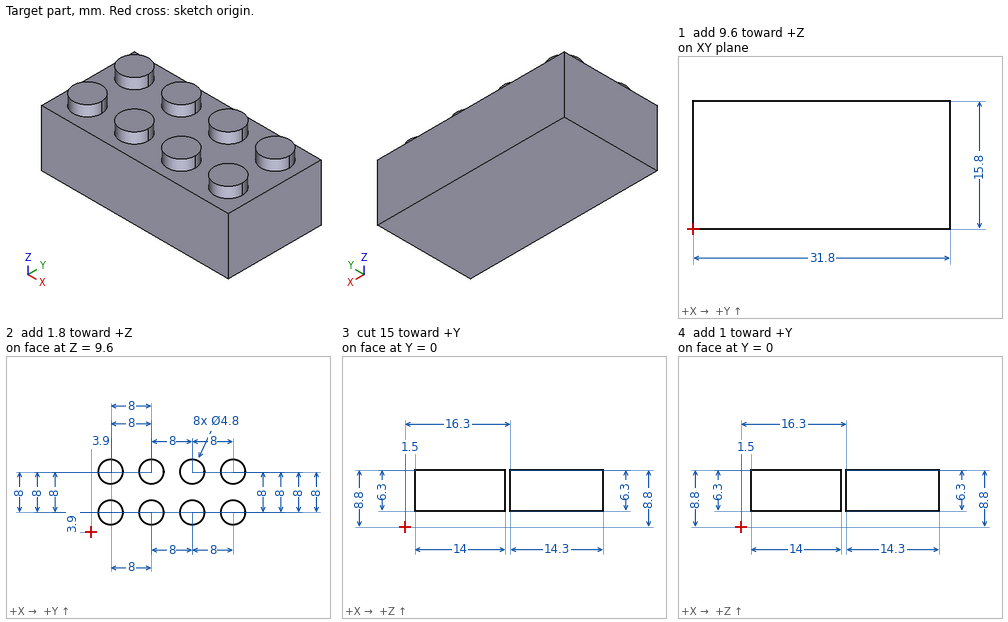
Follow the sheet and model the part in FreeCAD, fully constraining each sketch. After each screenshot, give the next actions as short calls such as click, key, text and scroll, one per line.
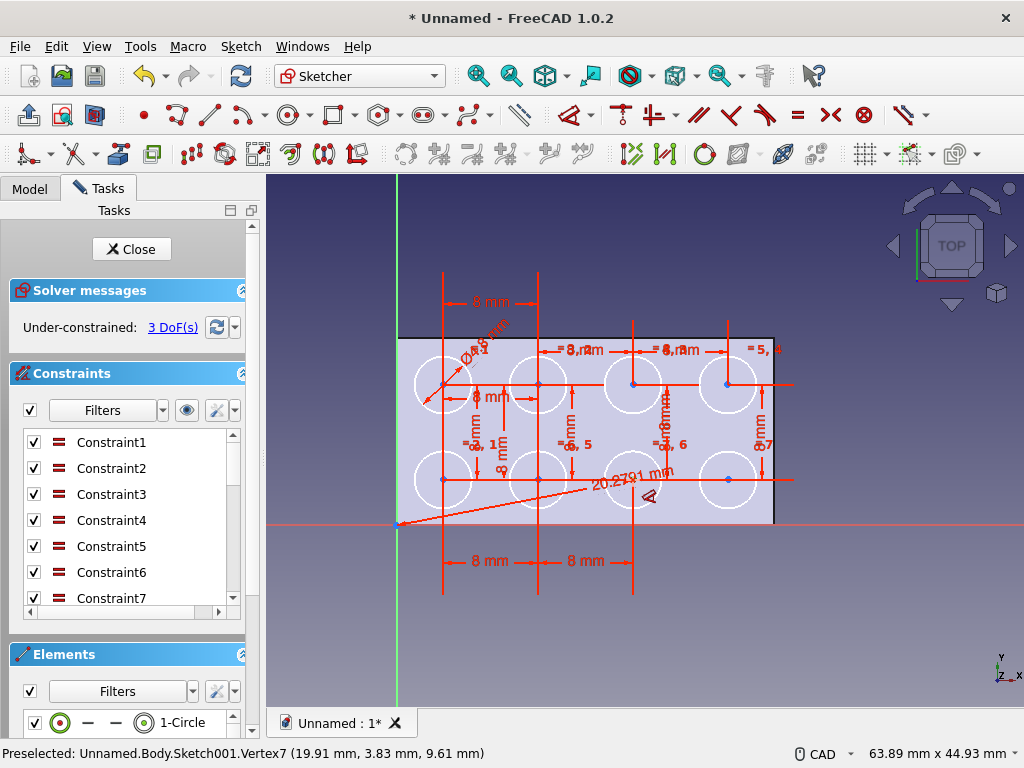
click(728, 480)
click(681, 562)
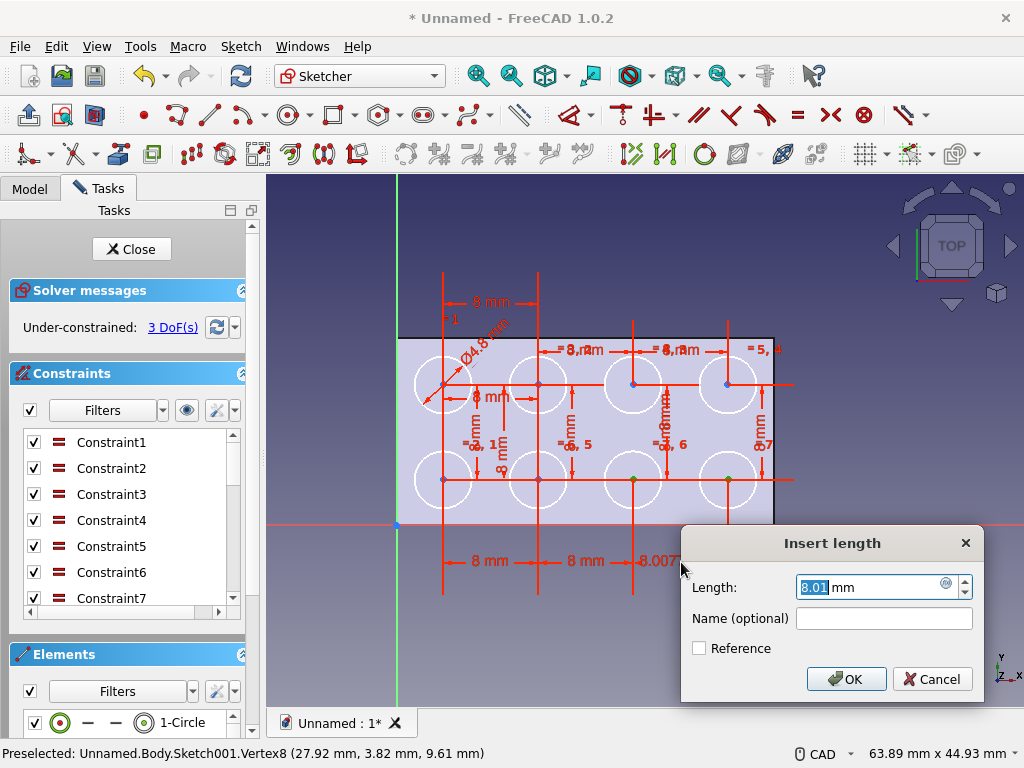
text(8)
key(Return)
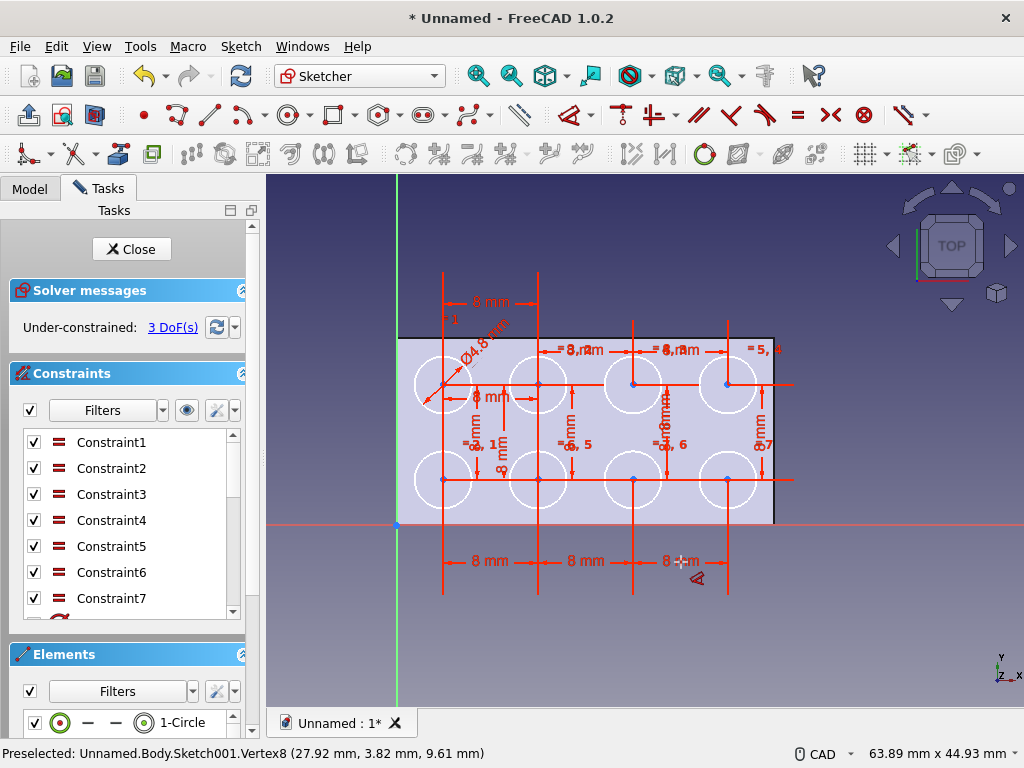
click(728, 385)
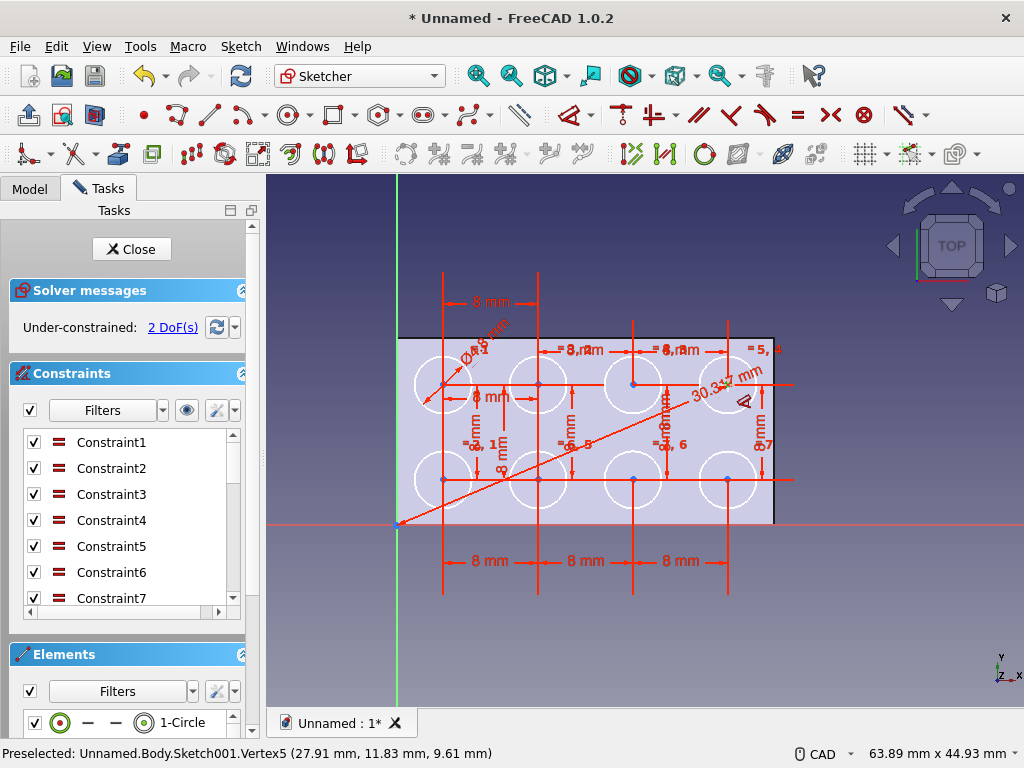
click(728, 480)
click(762, 411)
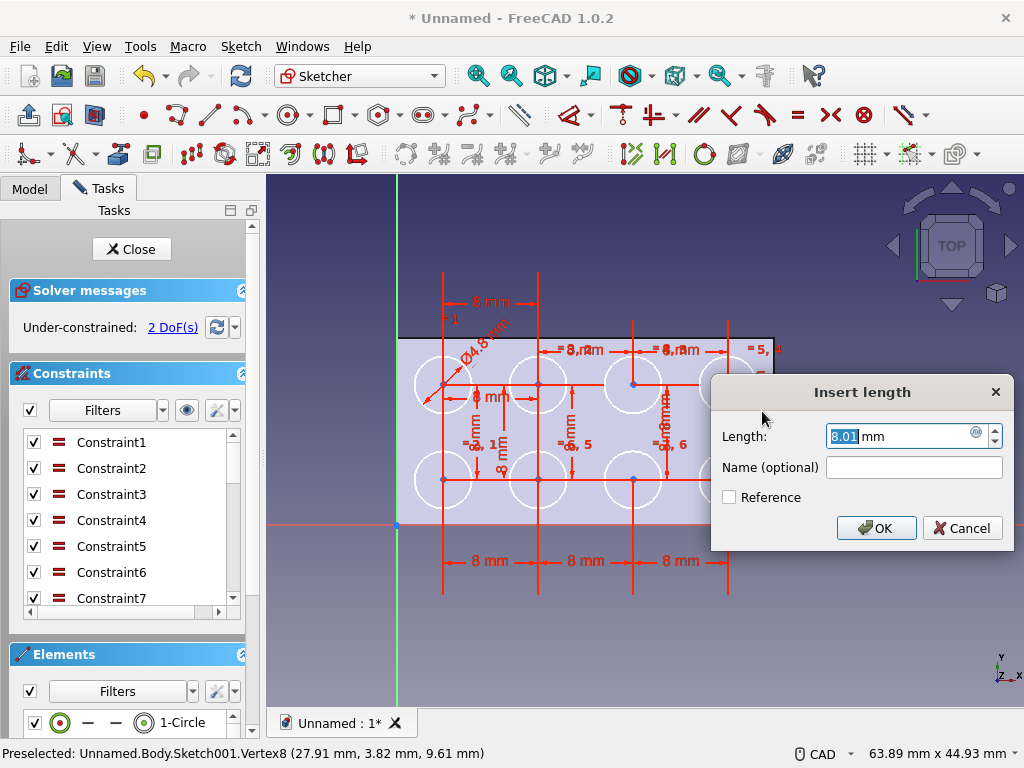
text(8)
key(Return)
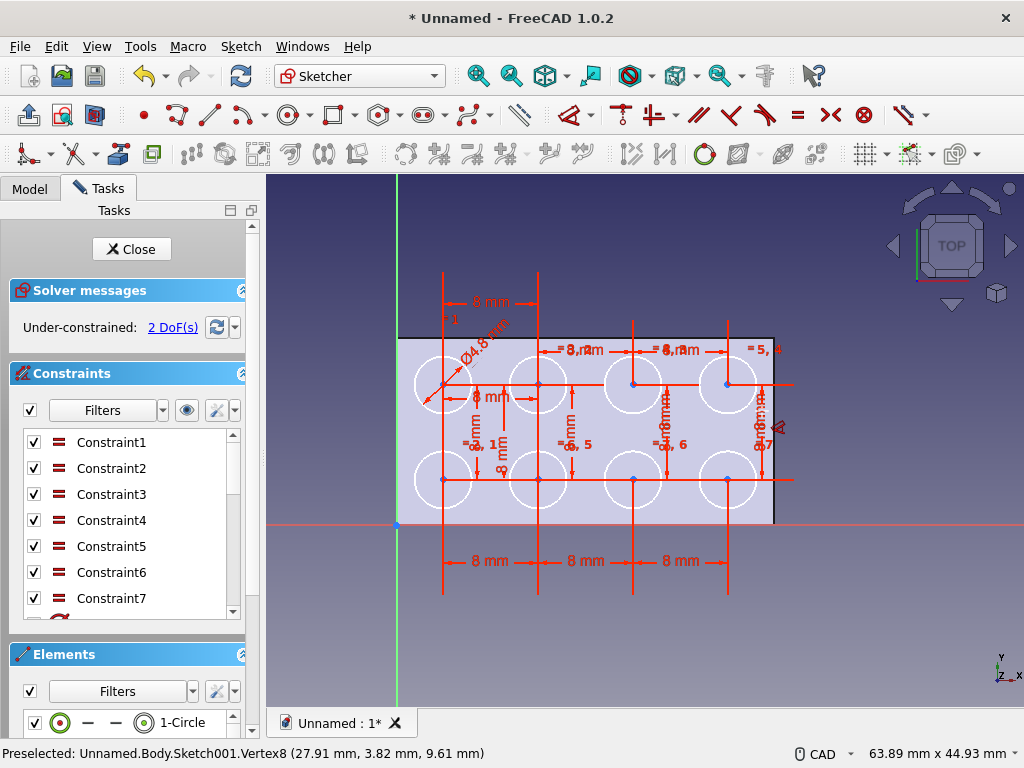
click(443, 385)
click(420, 559)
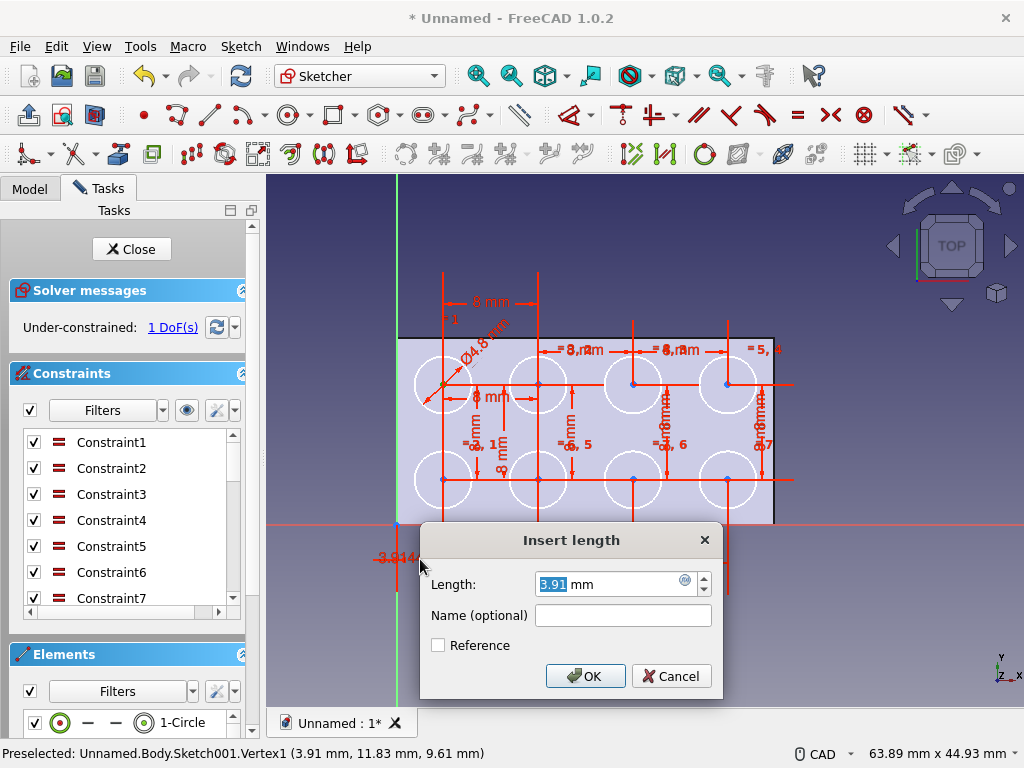
text(3.9)
key(Return)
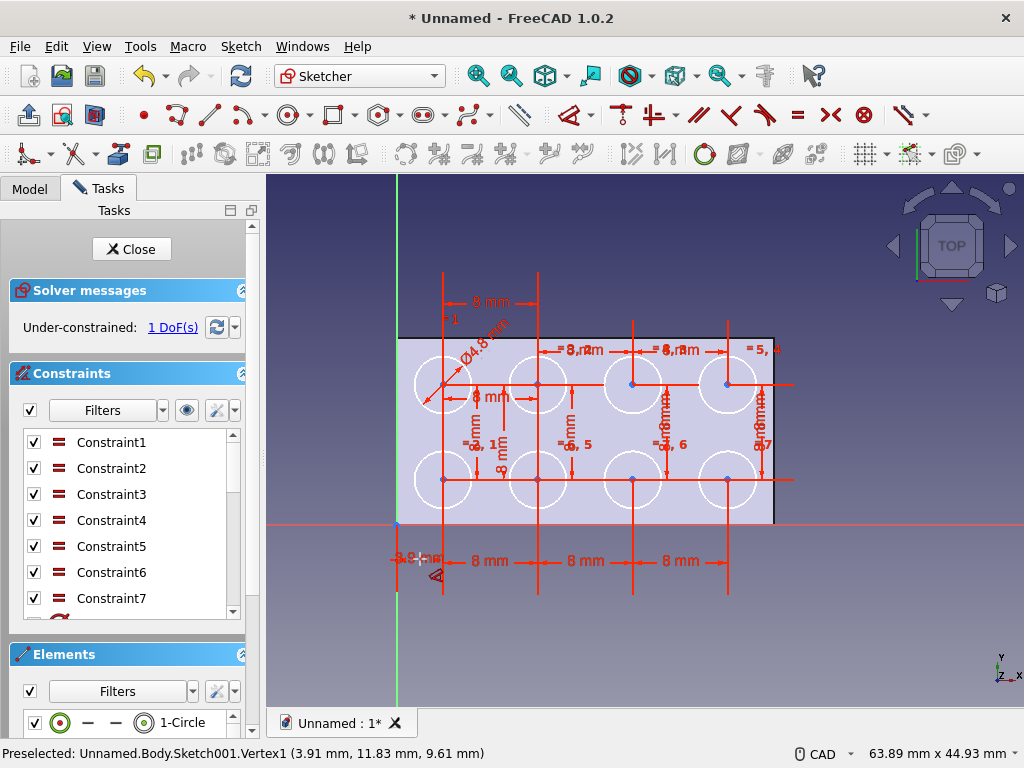
click(443, 480)
click(363, 503)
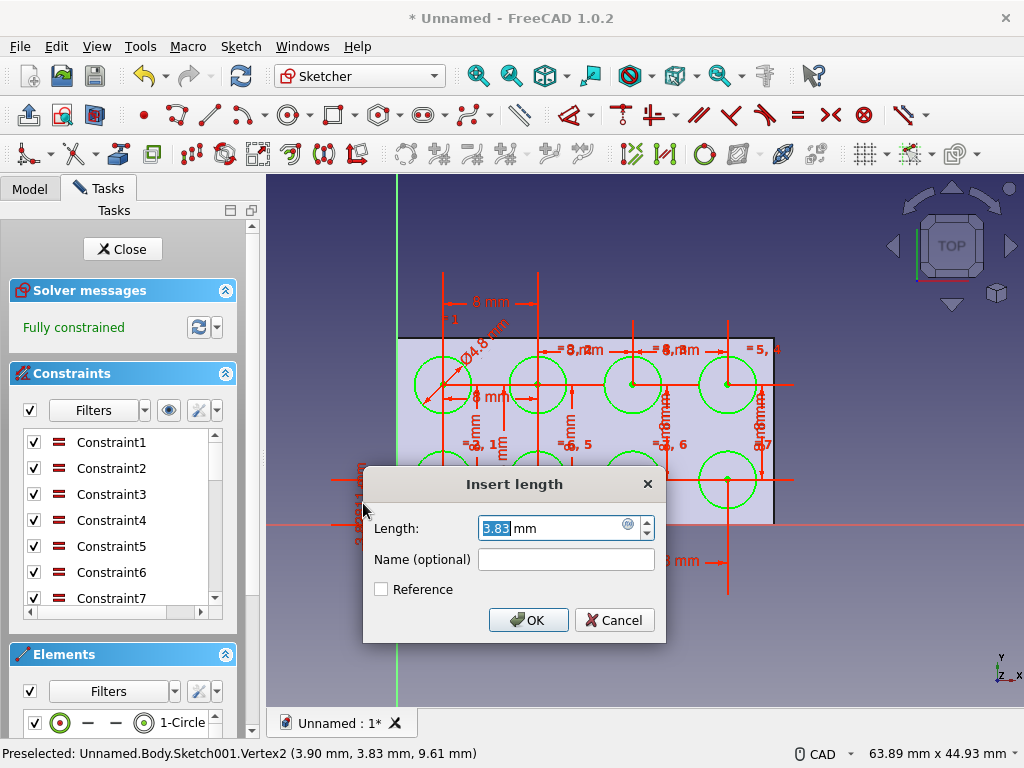
text(3.9)
key(Return)
key(Escape)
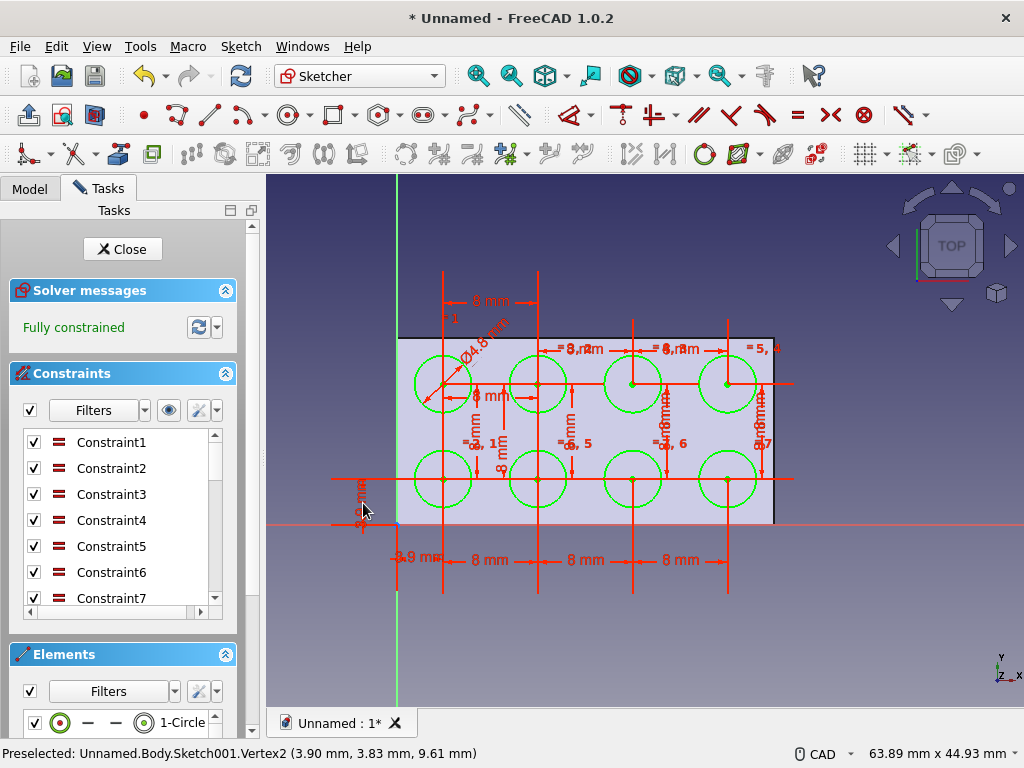
click(123, 249)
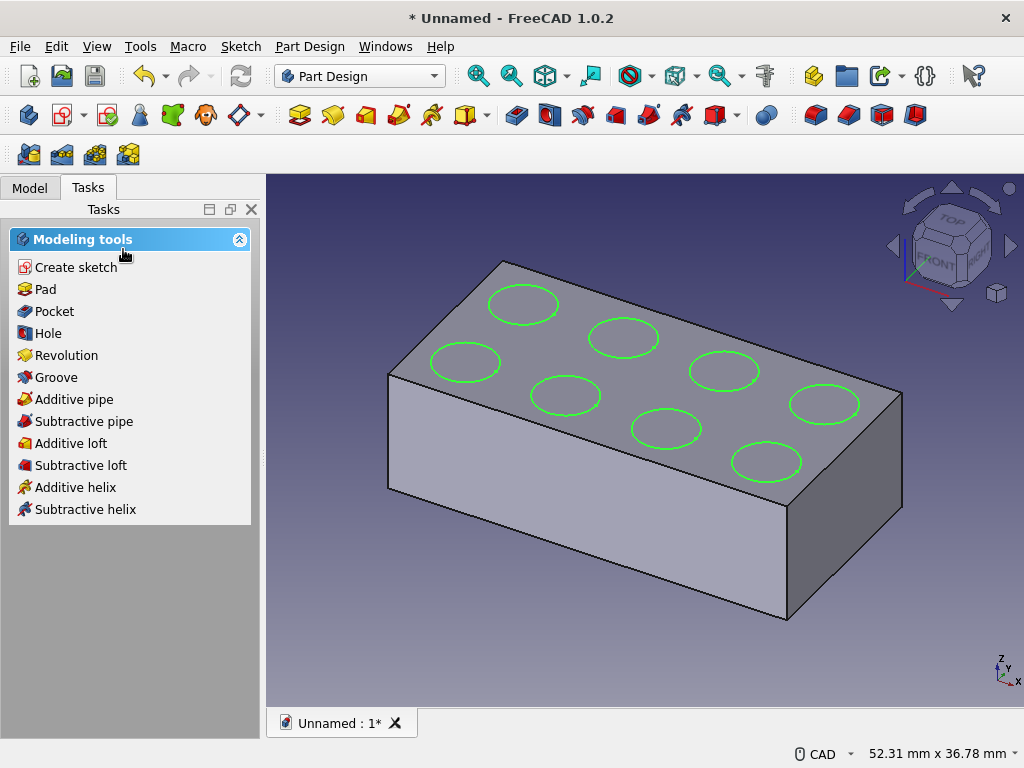
click(300, 116)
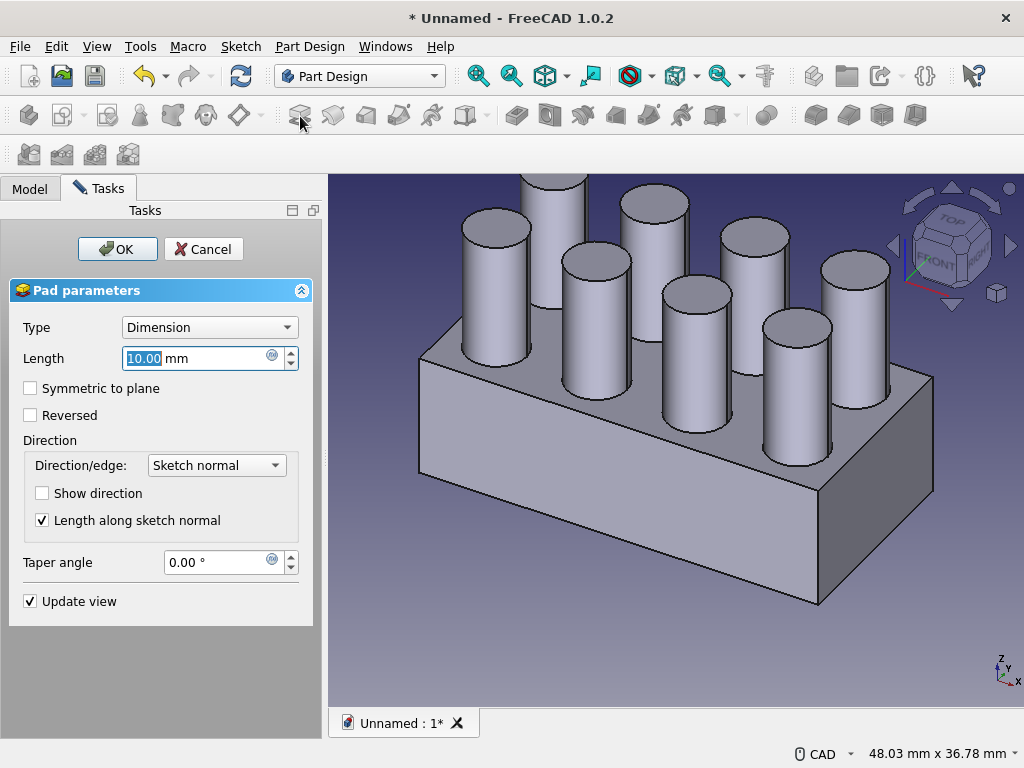
text(1.8)
key(Tab)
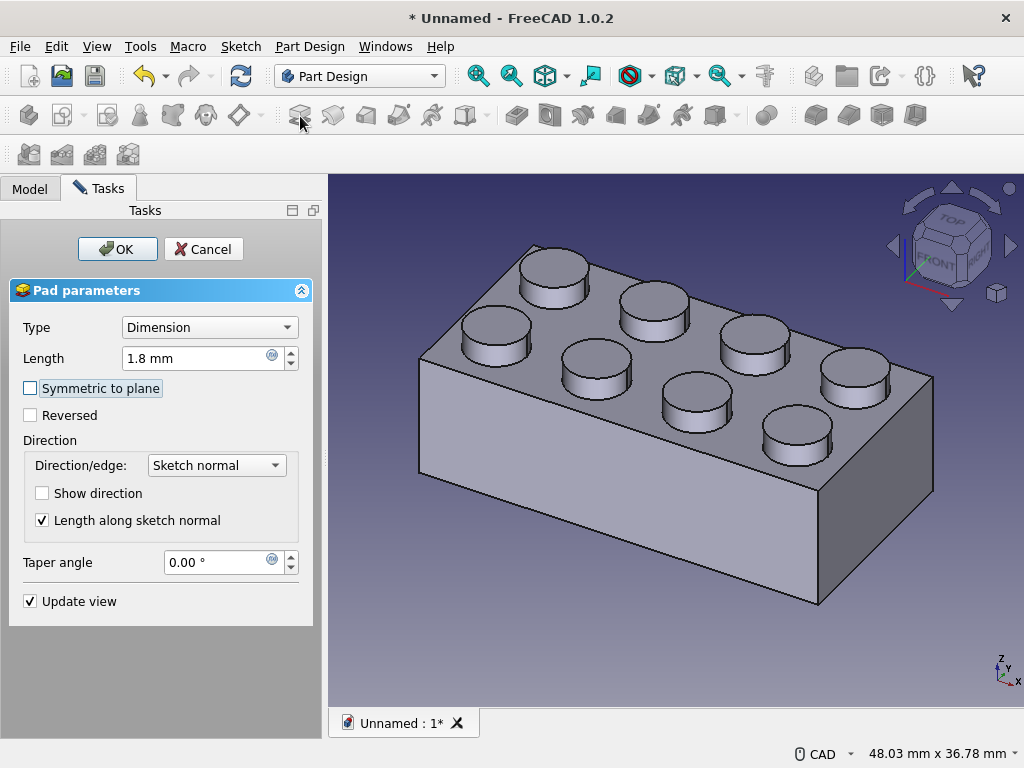
click(118, 249)